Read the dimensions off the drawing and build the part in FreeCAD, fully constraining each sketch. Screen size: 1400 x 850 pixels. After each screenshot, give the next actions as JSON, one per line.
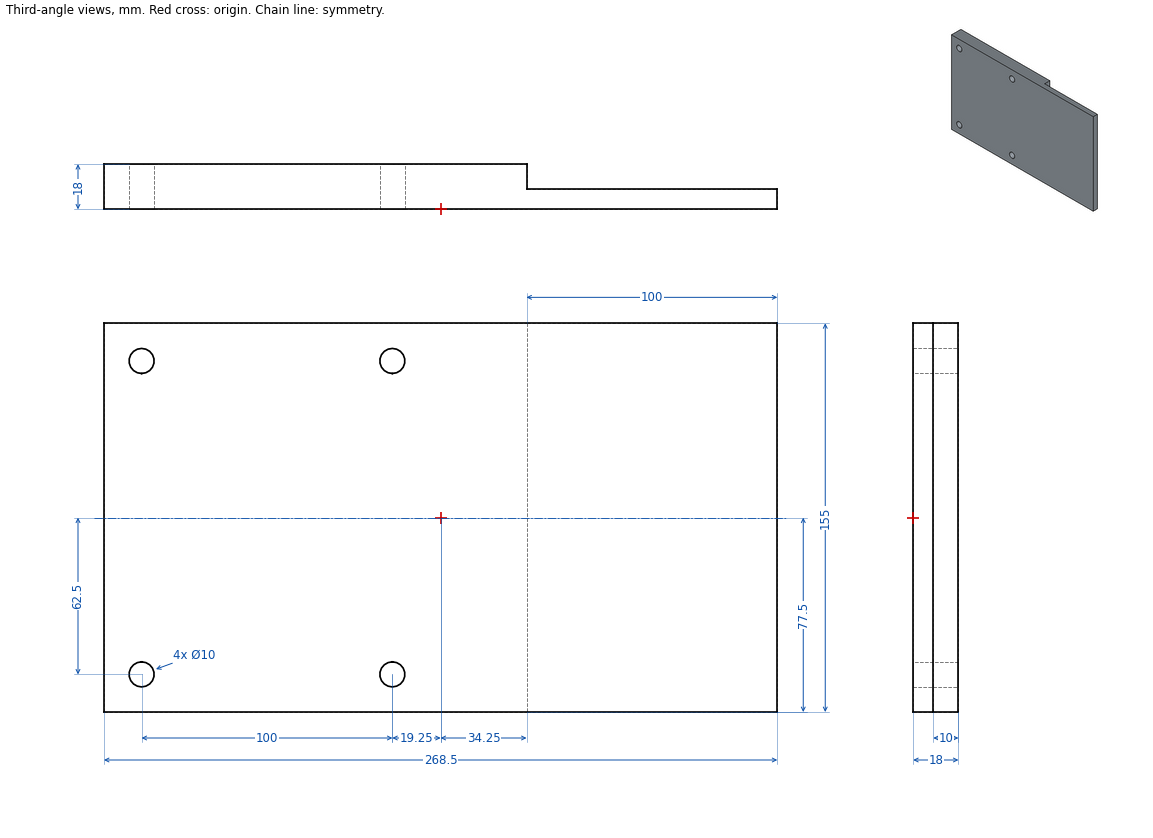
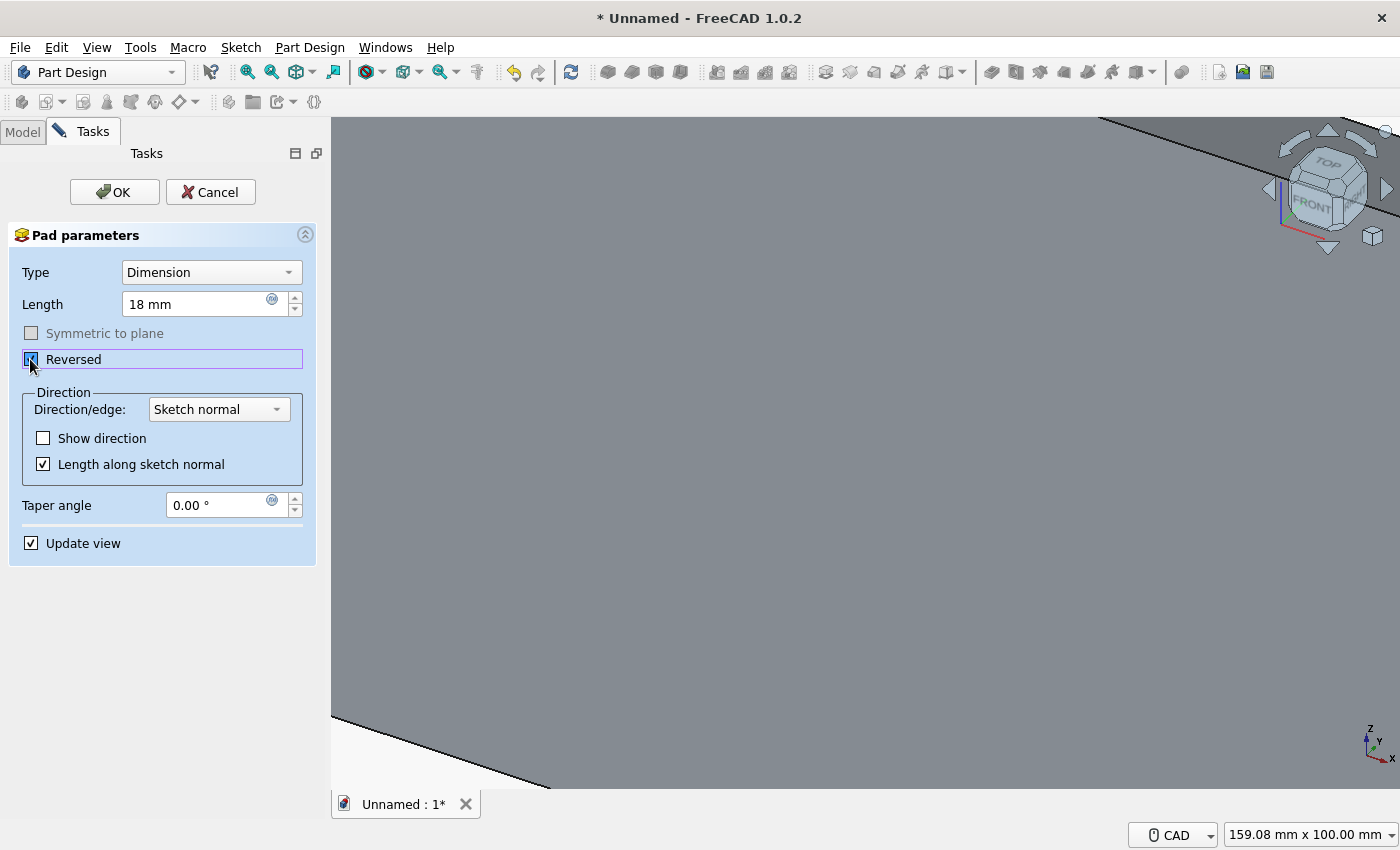
{"action": "left_click", "coordinate": [115, 192]}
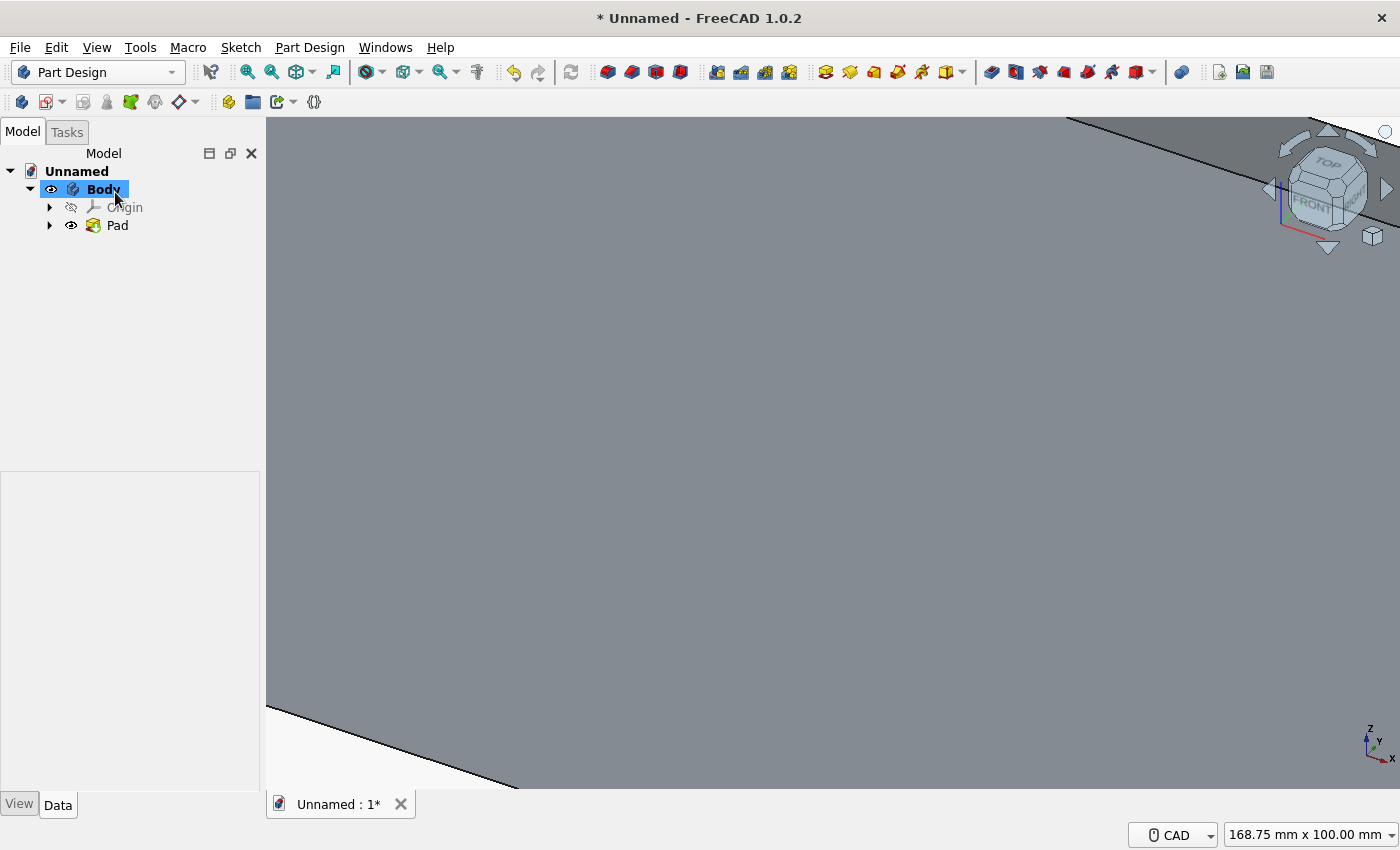
{"action": "key", "text": "v f"}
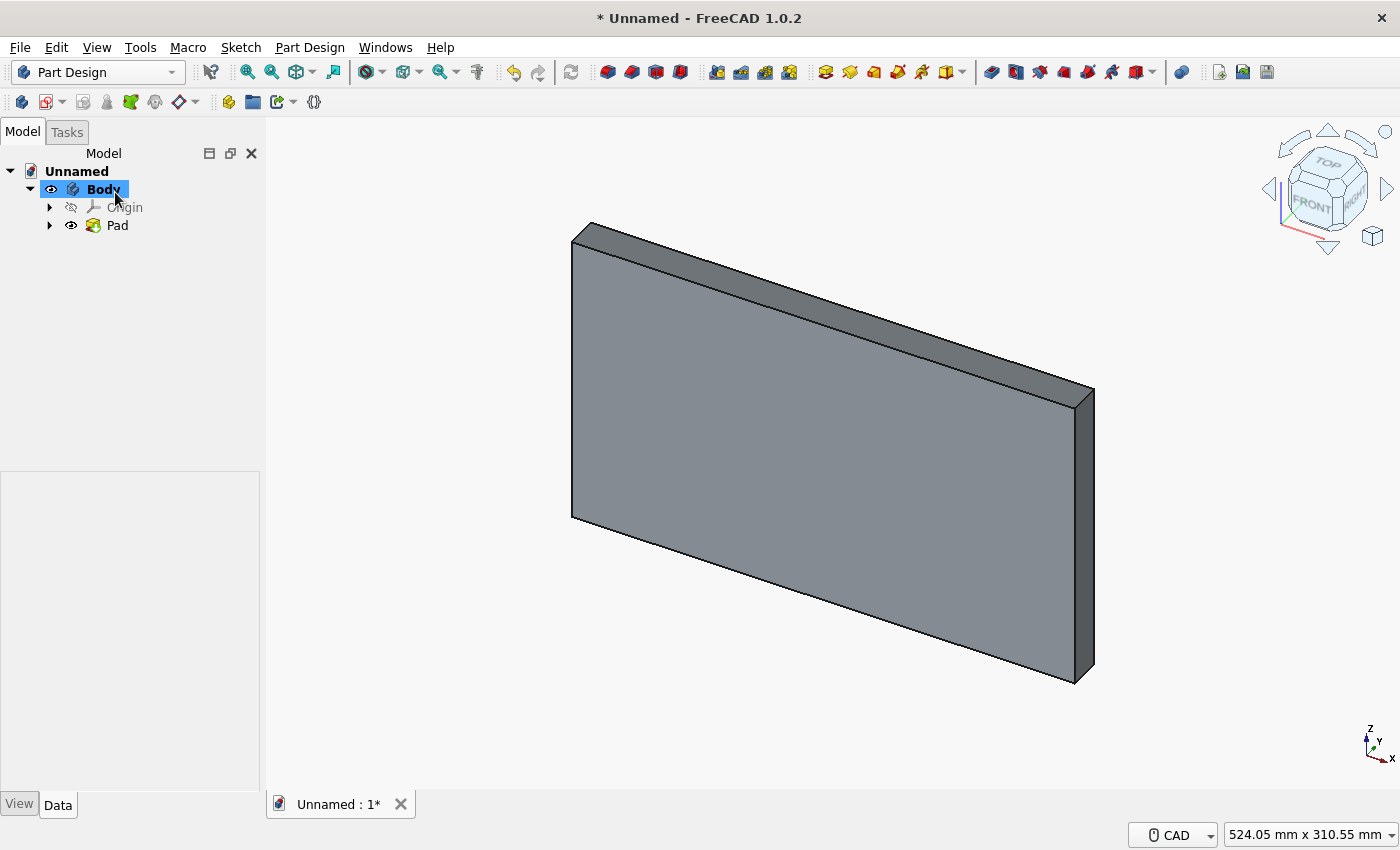
{"action": "key", "text": "4"}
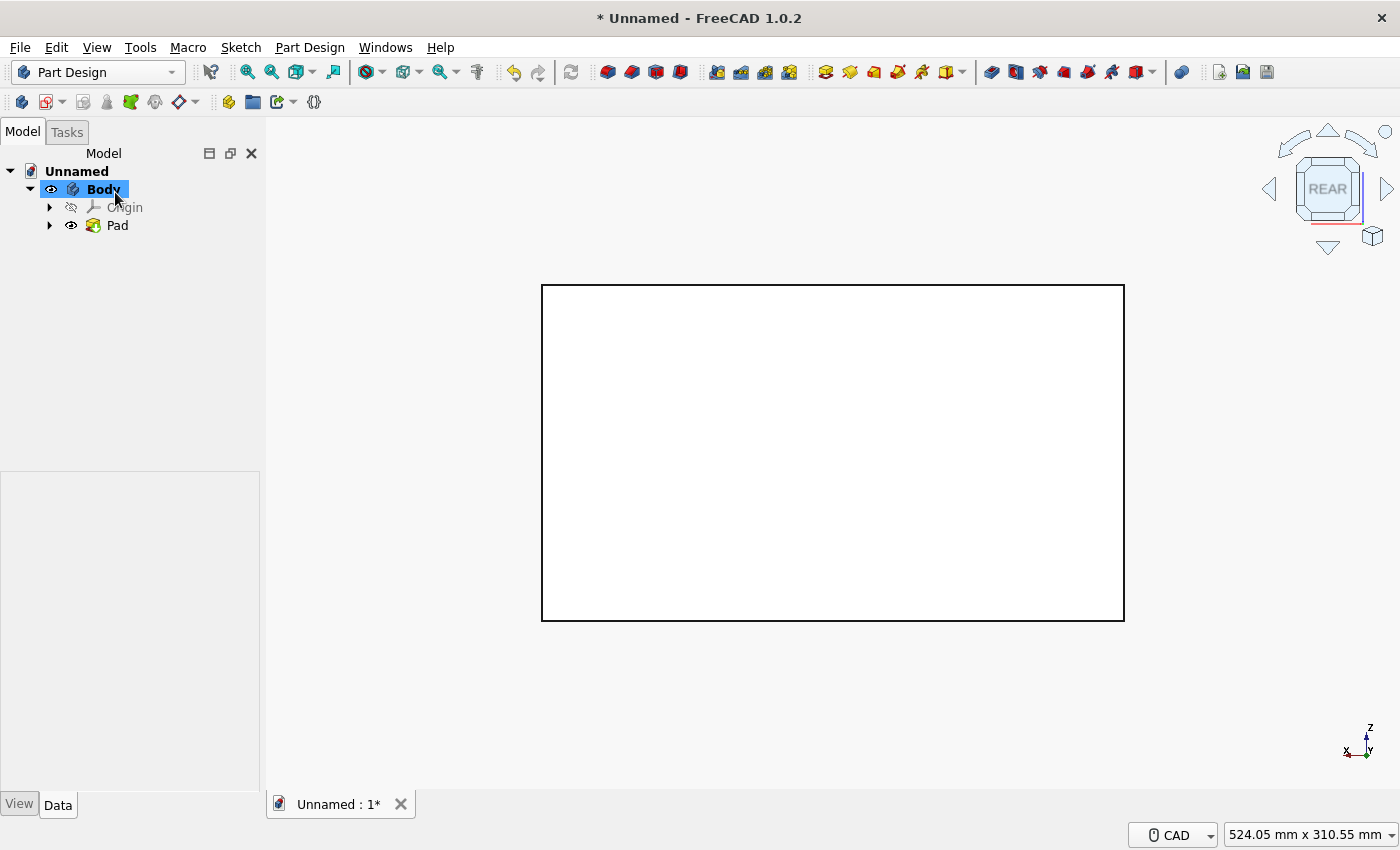
{"action": "left_click", "coordinate": [750, 452]}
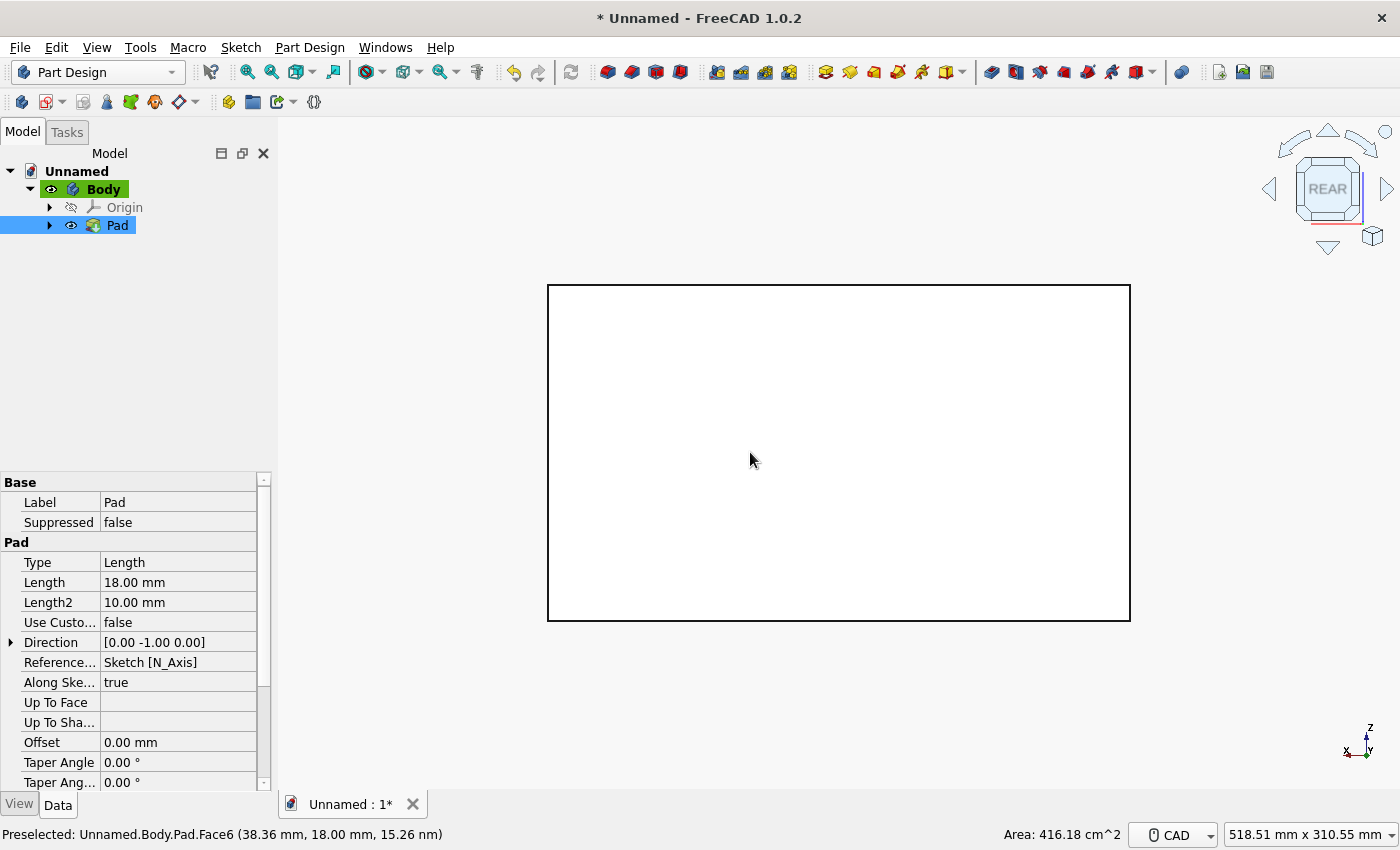
{"action": "left_click", "coordinate": [46, 102]}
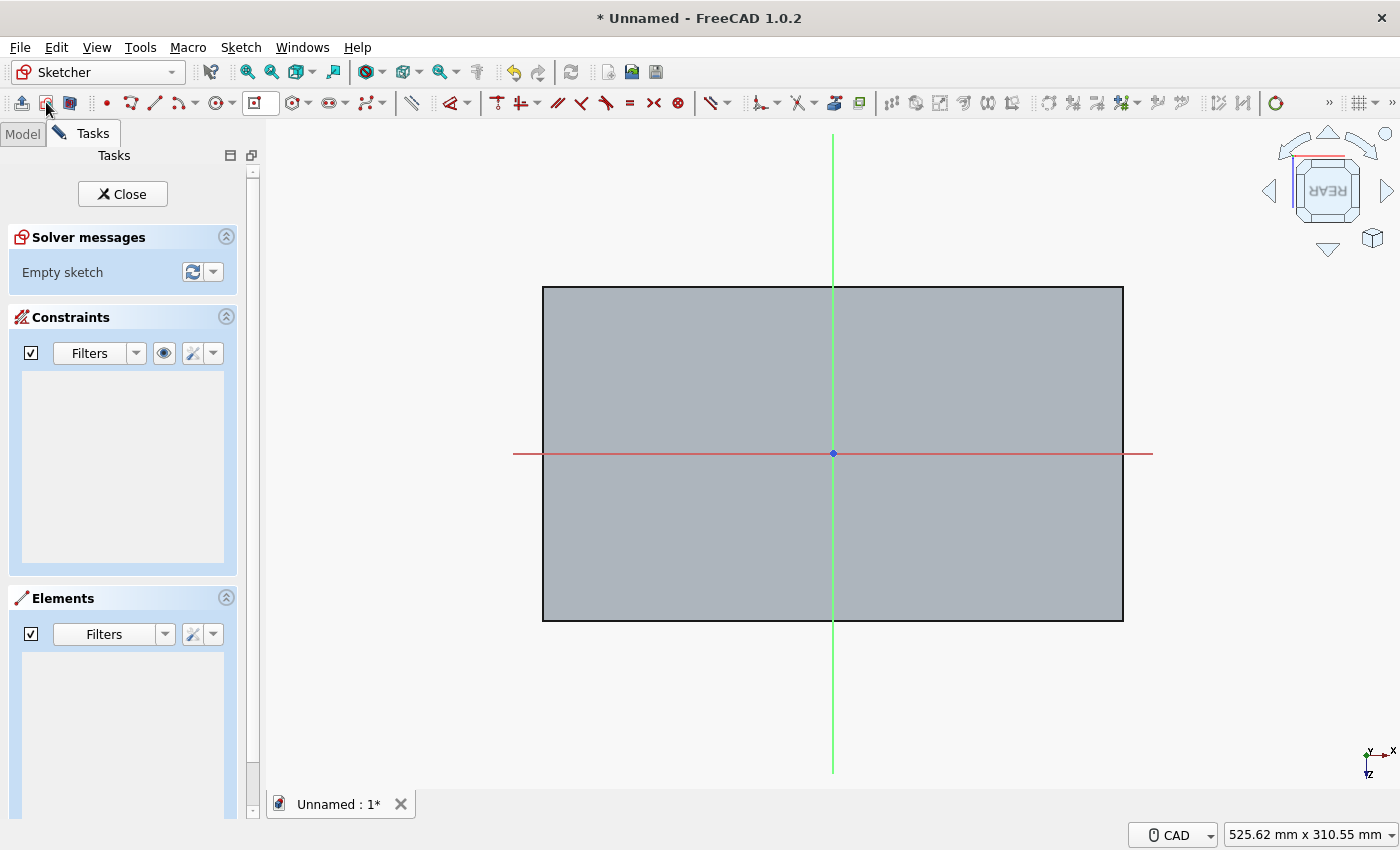
{"action": "scroll", "coordinate": [566, 454], "scroll_direction": "up", "scroll_amount": 2}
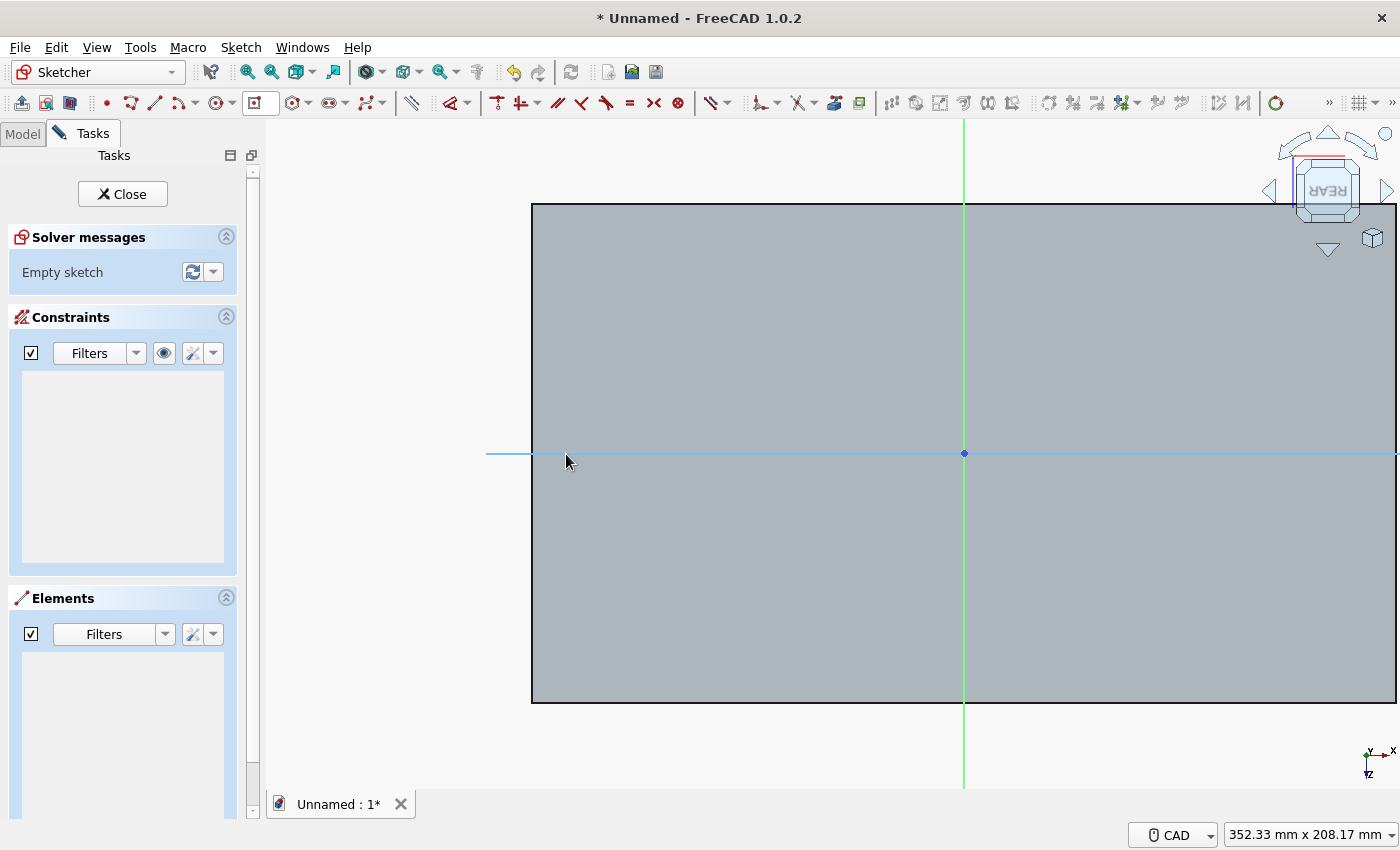
{"action": "left_click", "coordinate": [216, 104]}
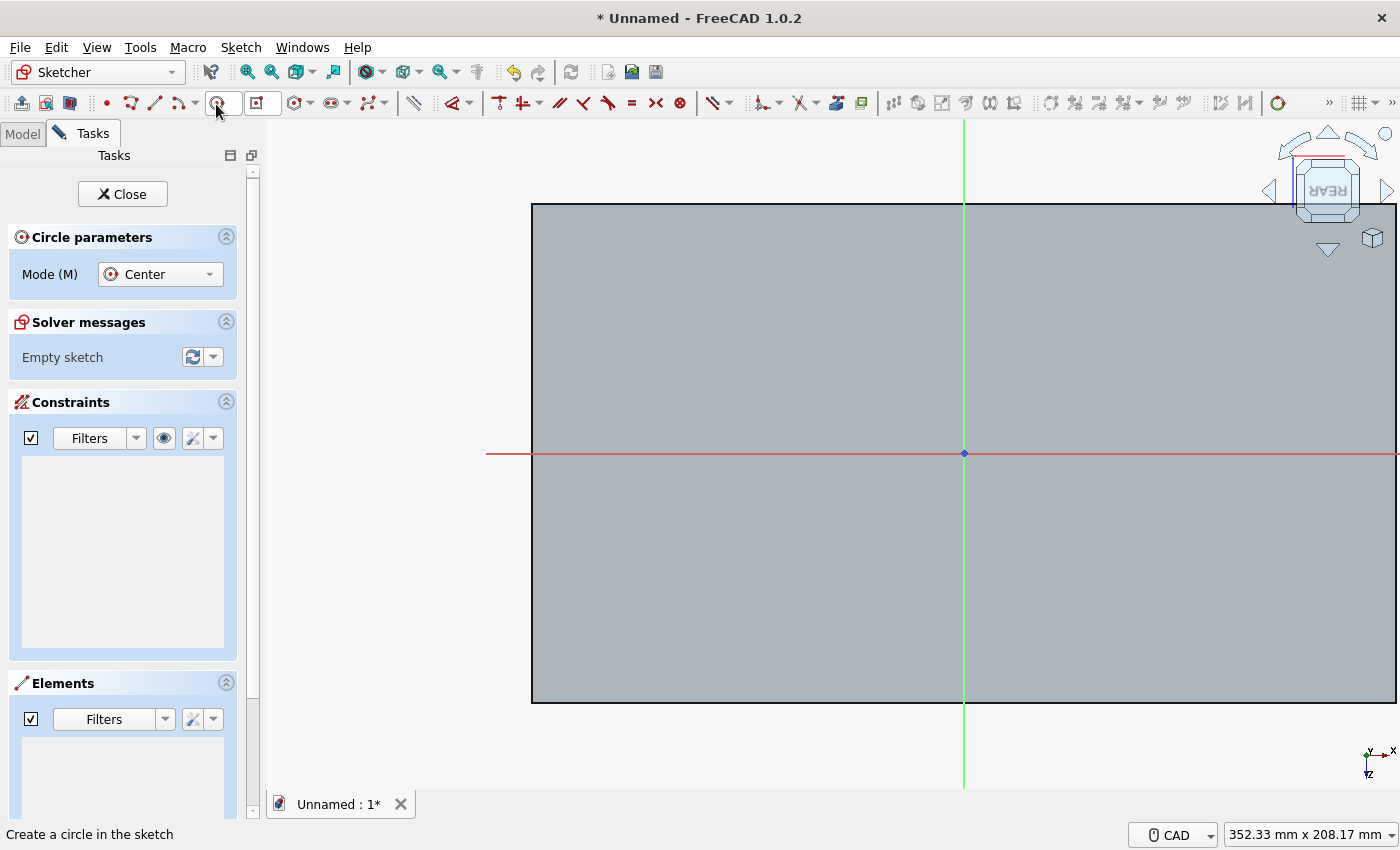
{"action": "scroll", "coordinate": [580, 253], "scroll_direction": "up", "scroll_amount": 2}